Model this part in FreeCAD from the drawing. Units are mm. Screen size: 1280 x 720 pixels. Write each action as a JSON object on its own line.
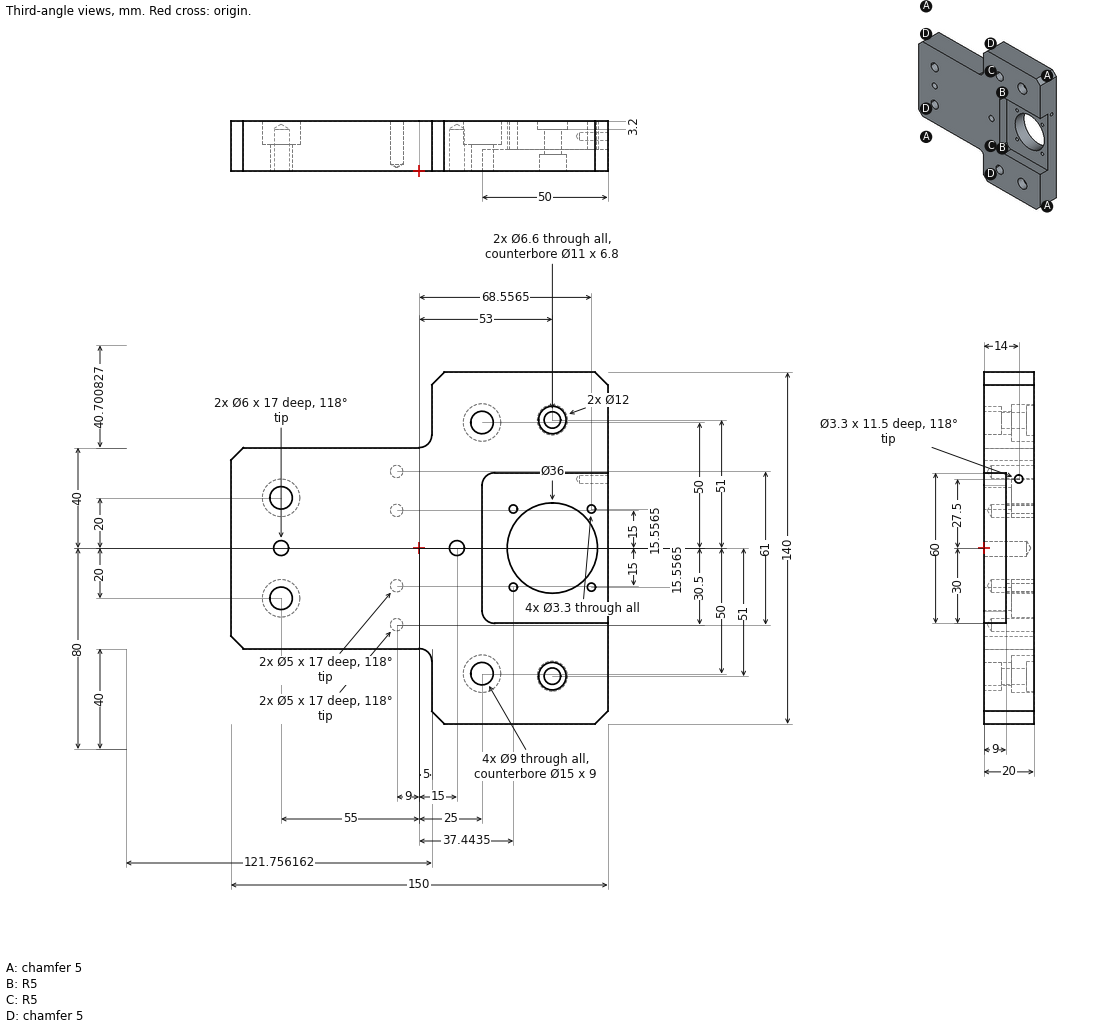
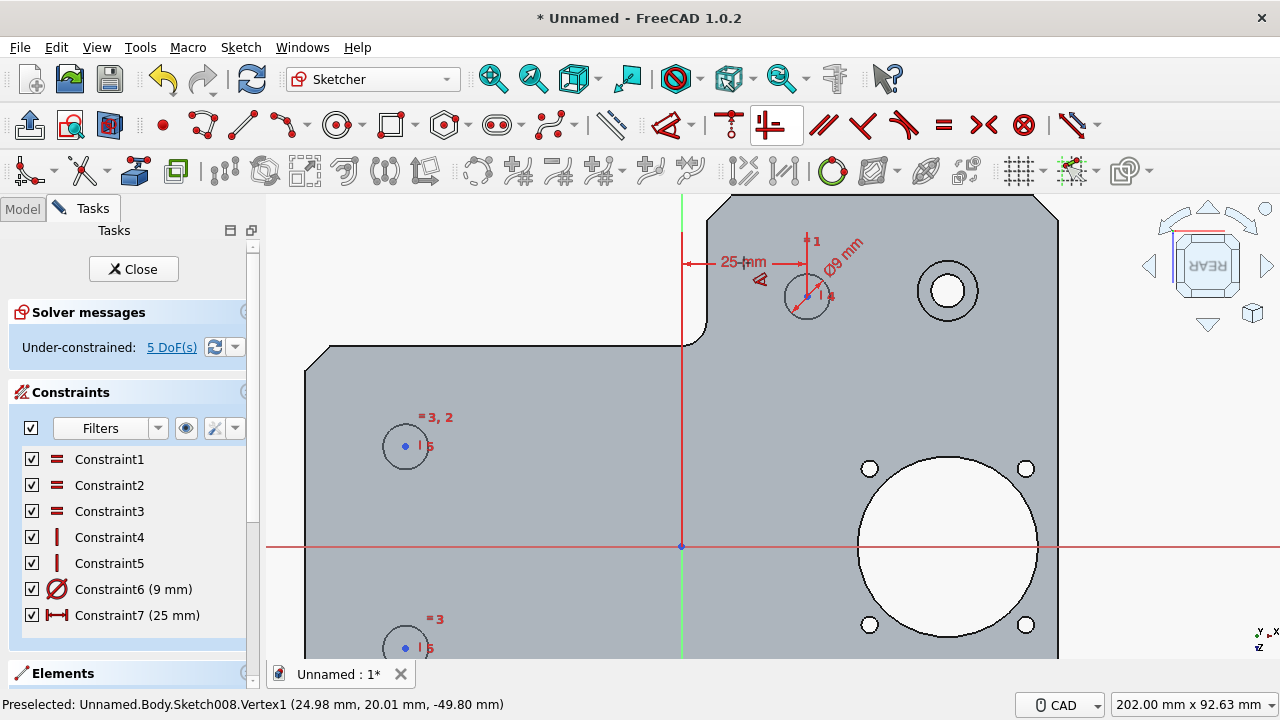
{"action": "left_click", "coordinate": [807, 297]}
{"action": "left_click", "coordinate": [841, 422]}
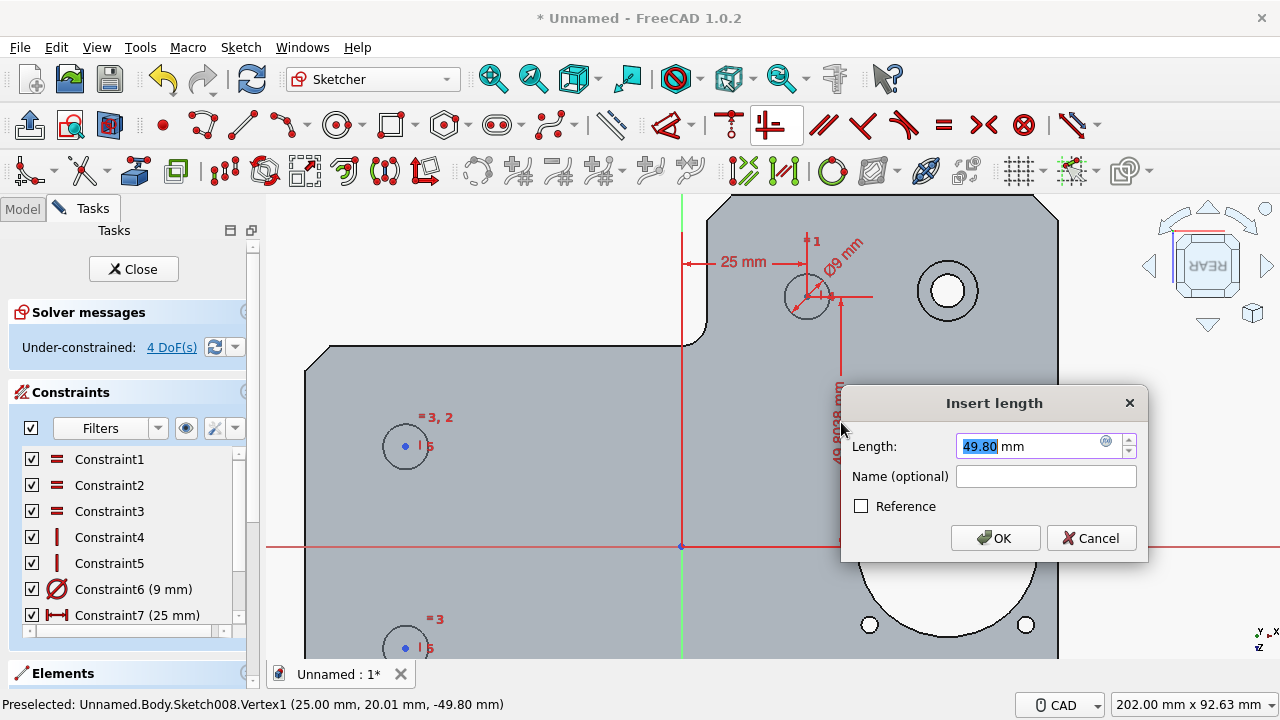
{"action": "type", "text": "50"}
{"action": "key", "text": "Return"}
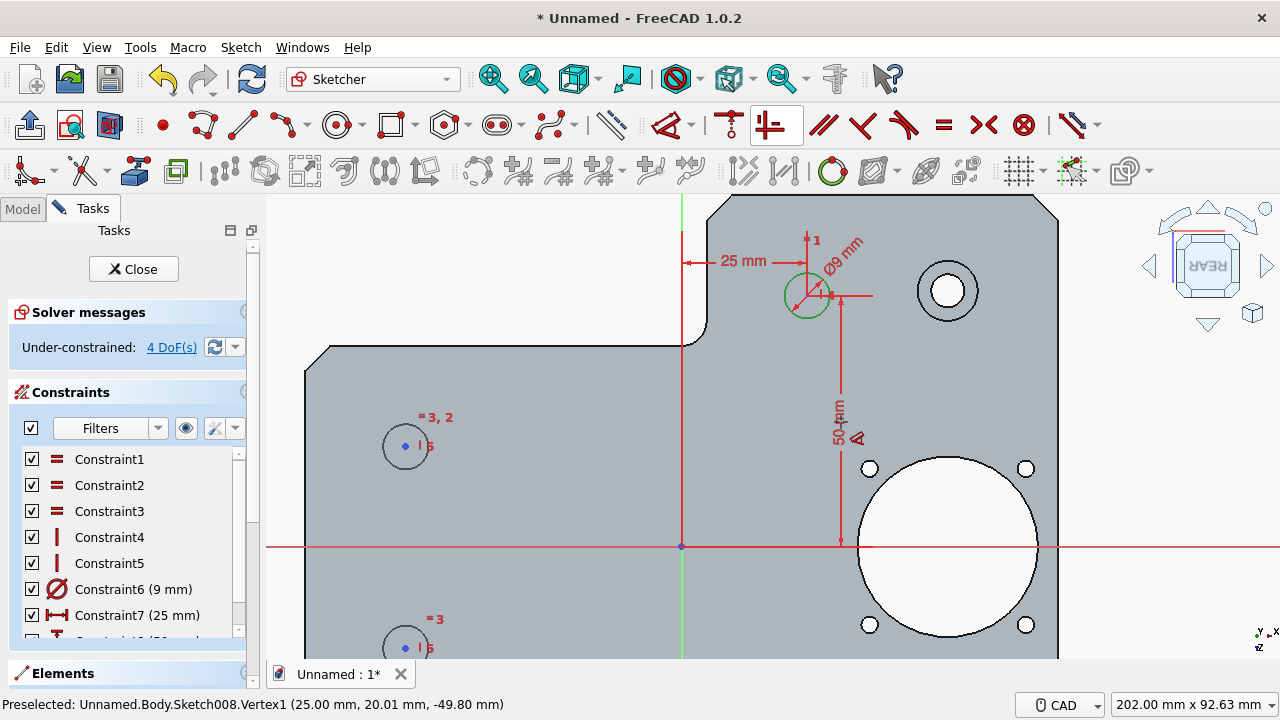
{"action": "scroll", "coordinate": [824, 280], "scroll_direction": "down", "scroll_amount": 3}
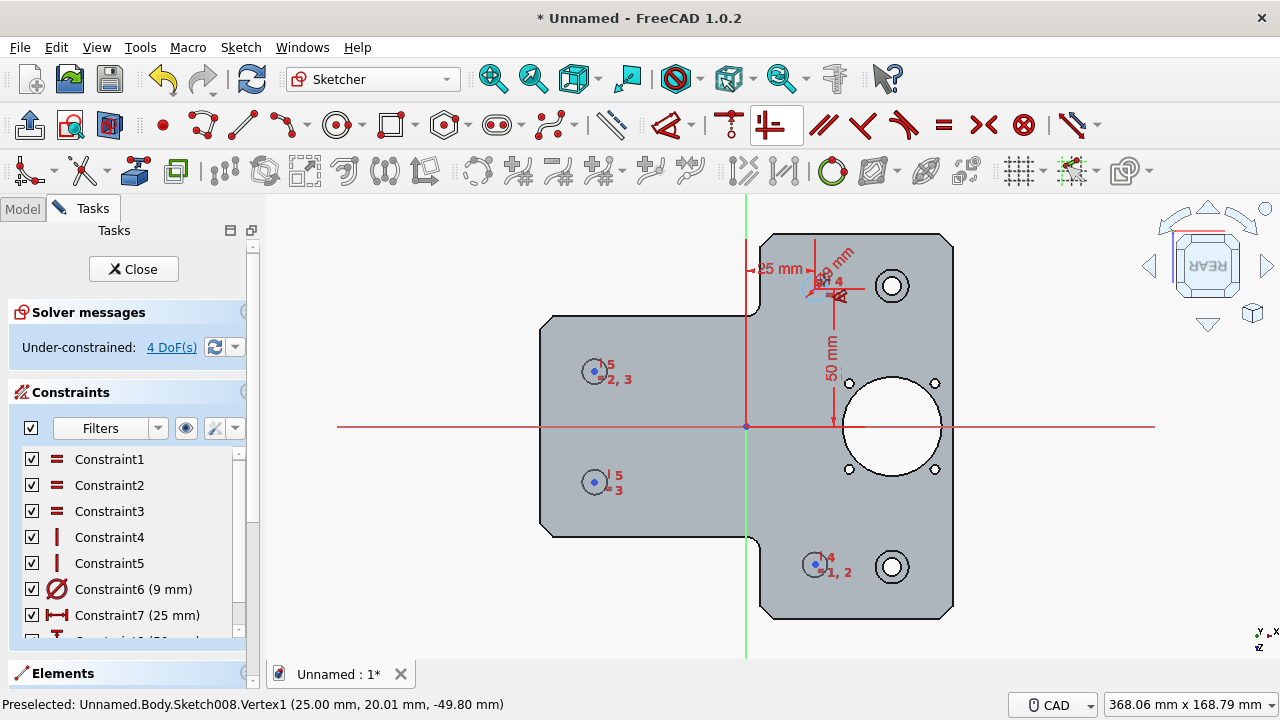
{"action": "left_click", "coordinate": [815, 565]}
{"action": "left_click", "coordinate": [849, 496]}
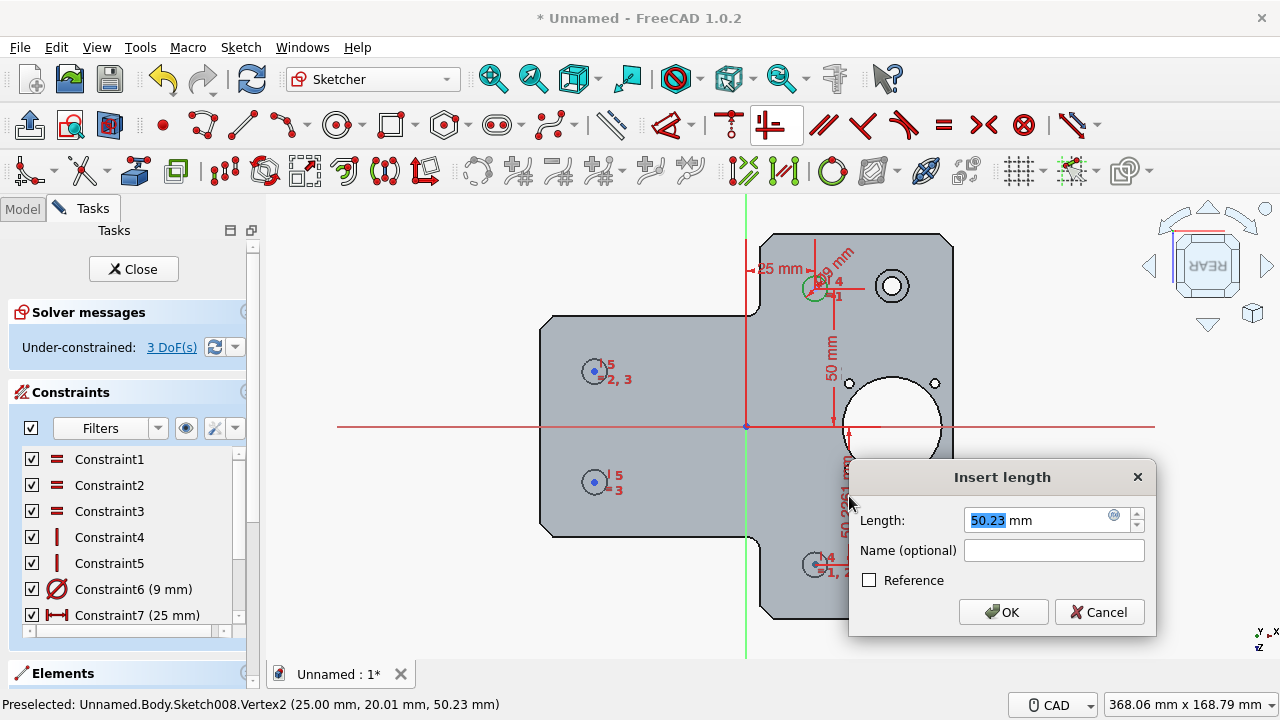
{"action": "type", "text": "50"}
{"action": "key", "text": "Return"}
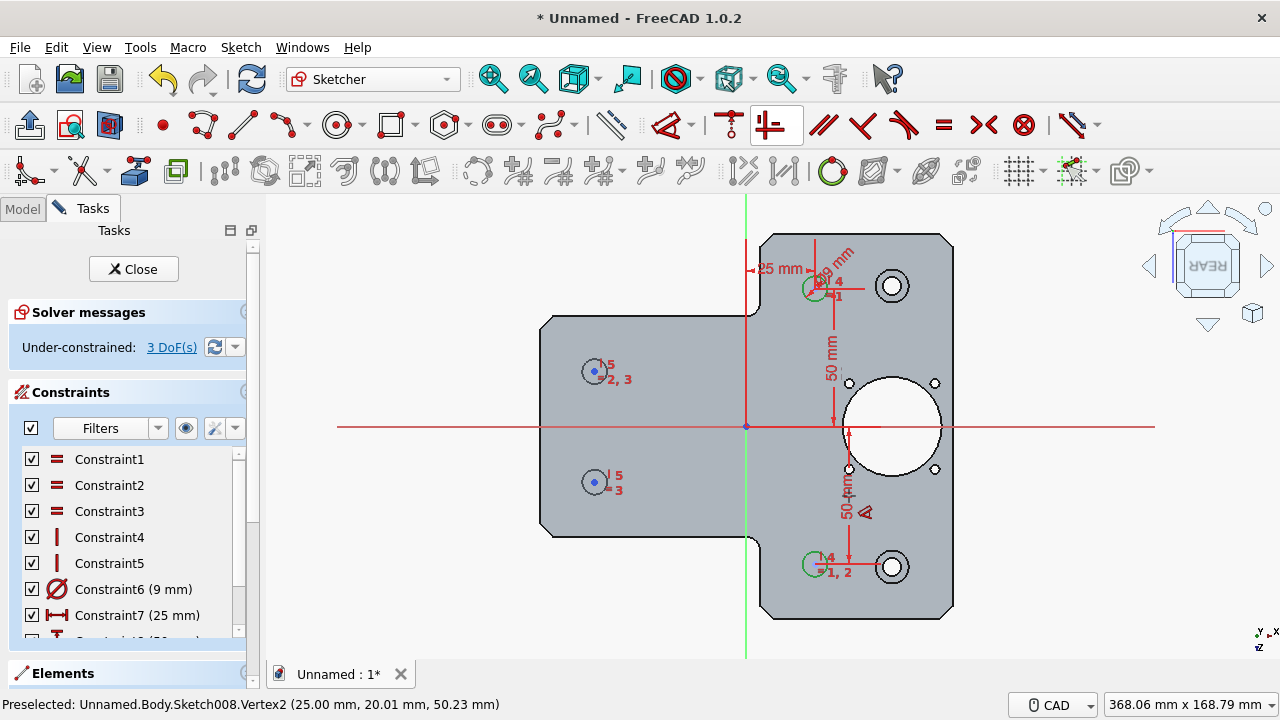
{"action": "left_click", "coordinate": [595, 372]}
{"action": "left_click", "coordinate": [670, 338]}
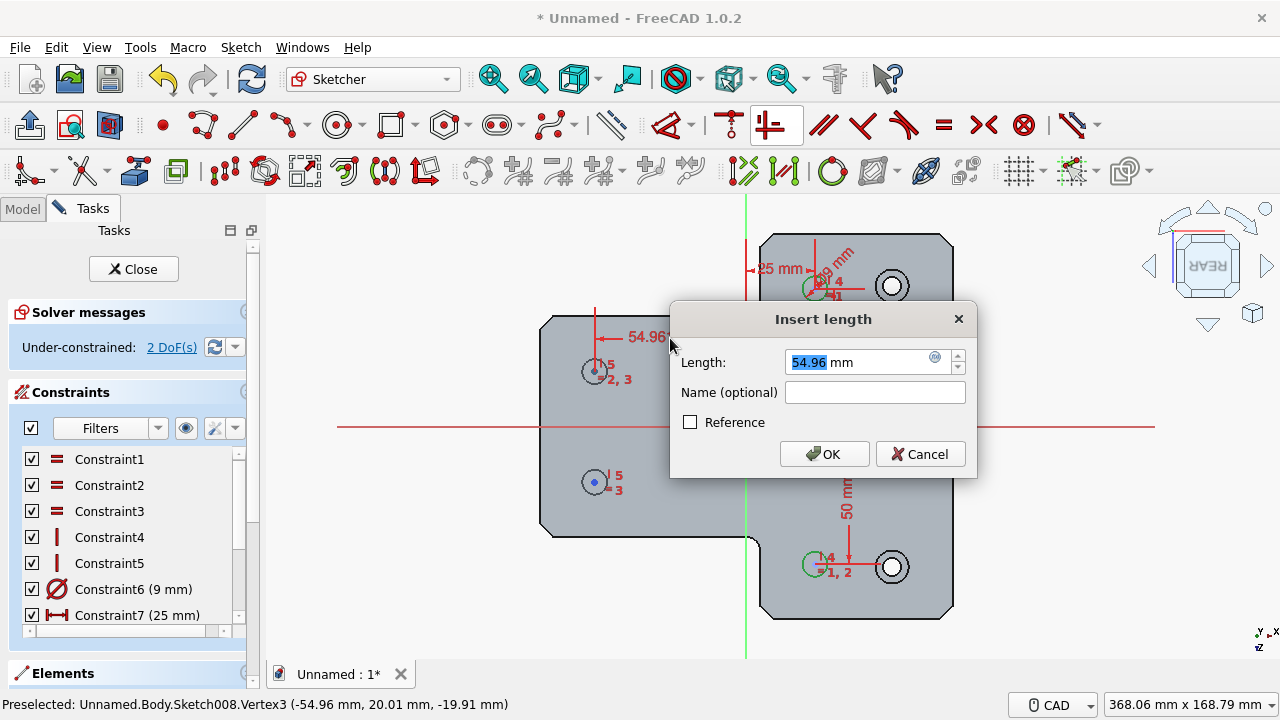
{"action": "type", "text": "55"}
{"action": "key", "text": "Return"}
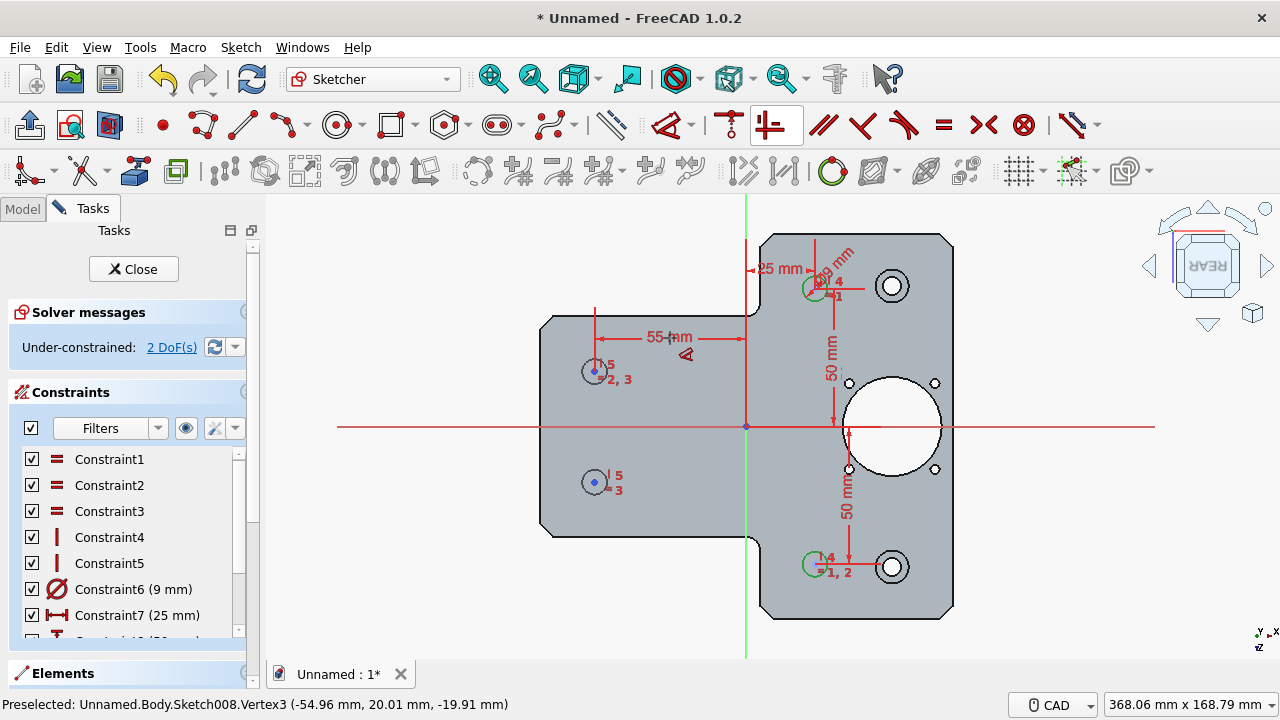
{"action": "left_click", "coordinate": [595, 372]}
{"action": "left_click", "coordinate": [561, 399]}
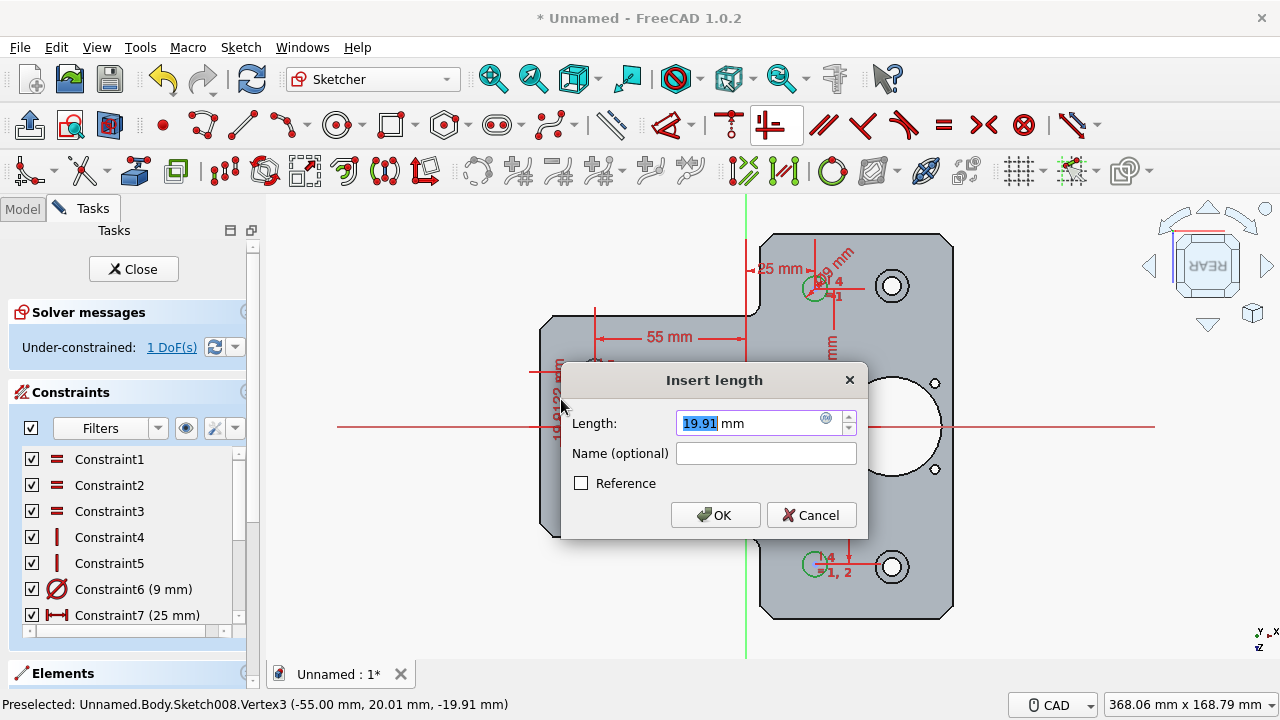
{"action": "type", "text": "20"}
{"action": "key", "text": "Return"}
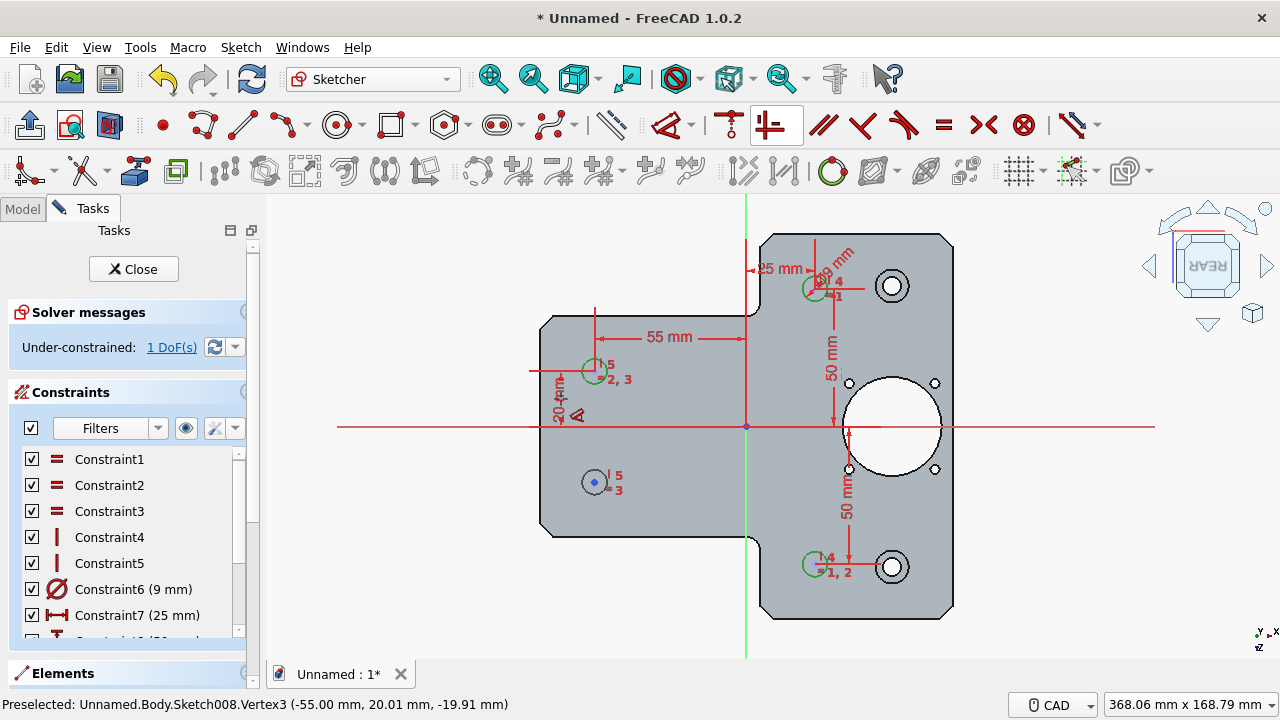
{"action": "left_click", "coordinate": [595, 482]}
{"action": "left_click", "coordinate": [561, 454]}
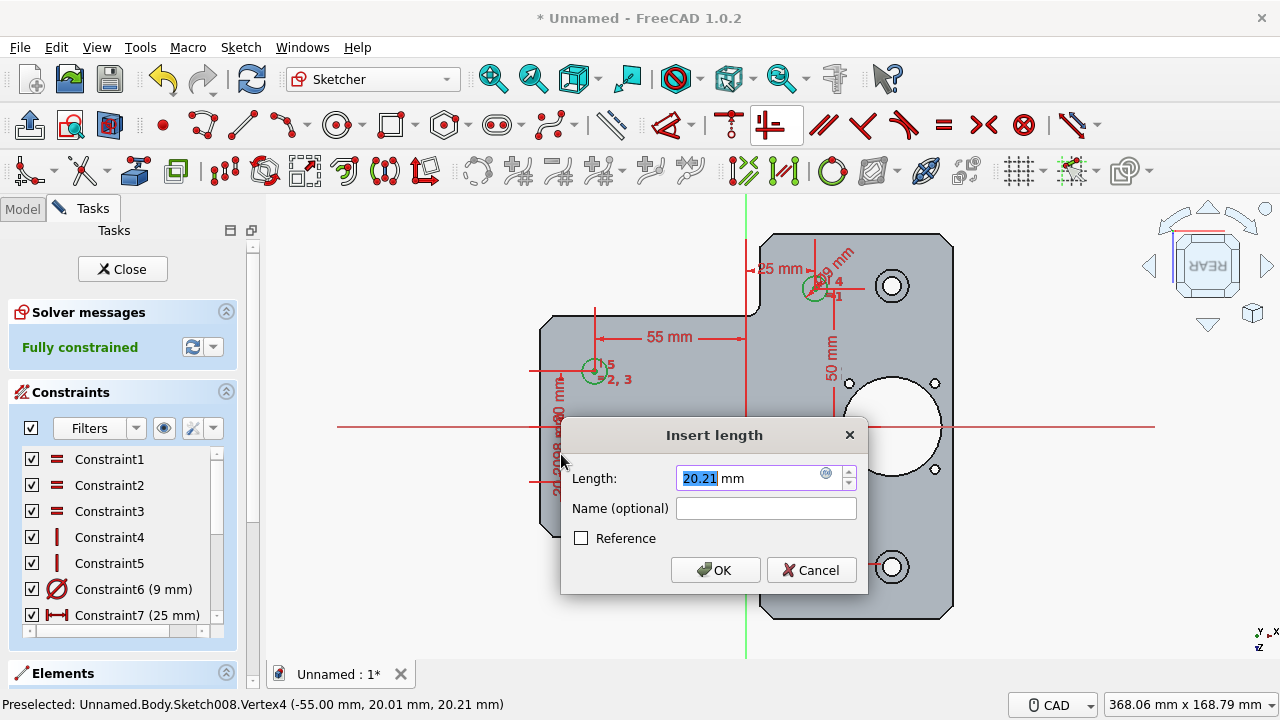
{"action": "type", "text": "20"}
{"action": "key", "text": "Return"}
{"action": "key", "text": "Escape"}